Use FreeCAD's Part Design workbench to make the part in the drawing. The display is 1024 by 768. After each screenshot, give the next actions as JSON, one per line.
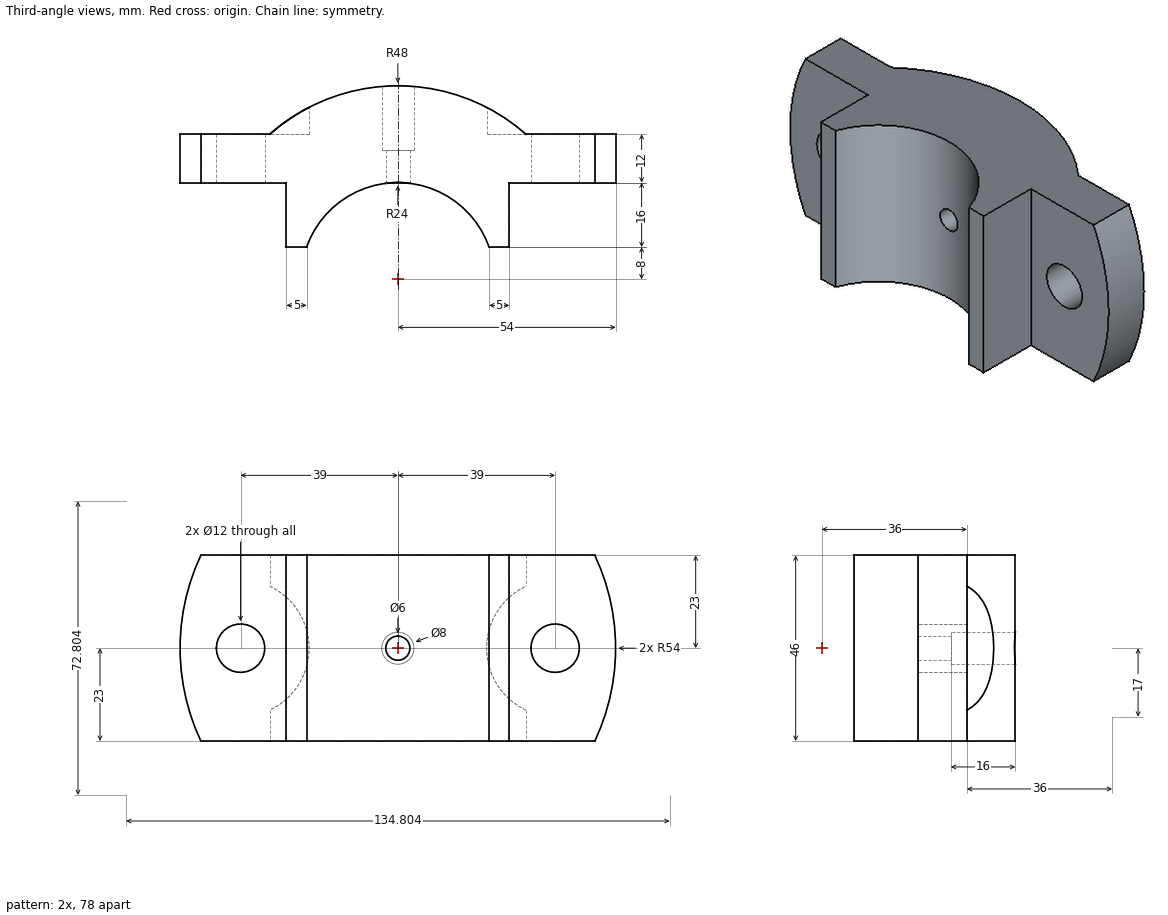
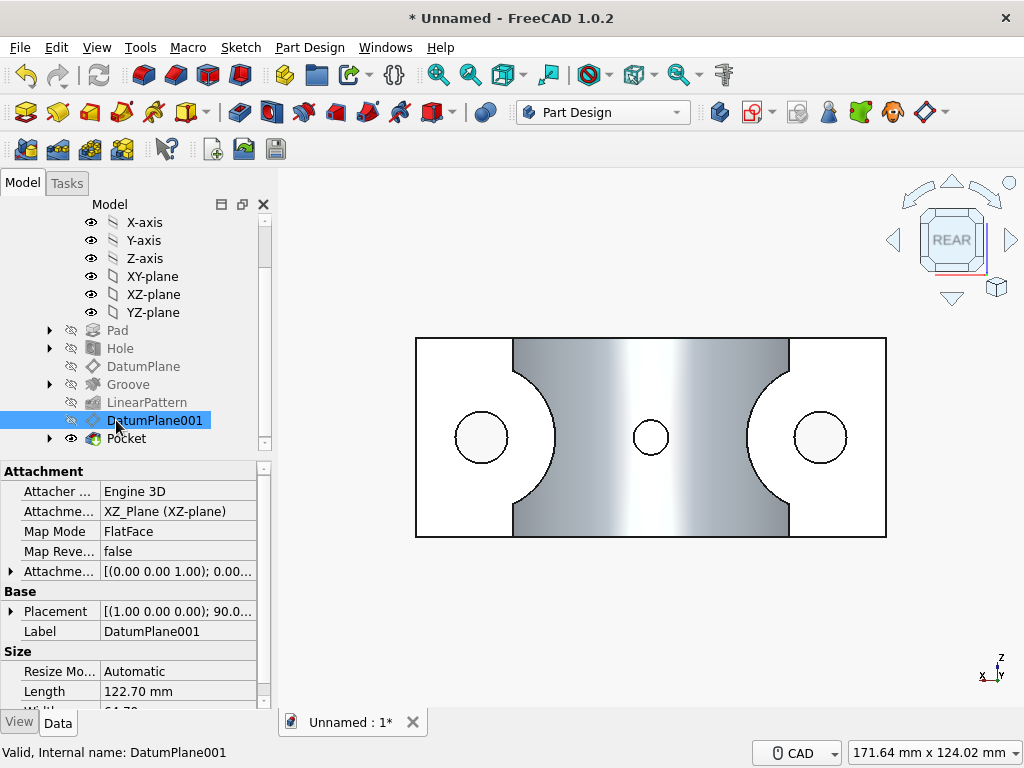
{"action": "scroll", "coordinate": [160, 326], "scroll_direction": "down", "scroll_amount": 3}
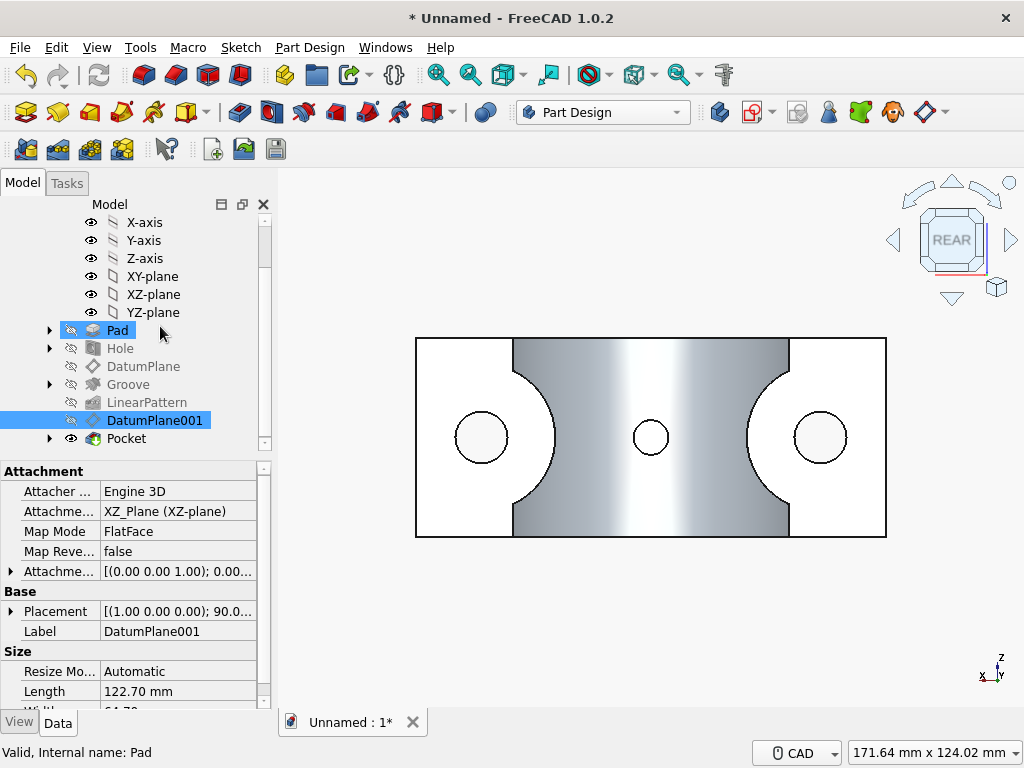
{"action": "scroll", "coordinate": [160, 326], "scroll_direction": "up", "scroll_amount": 15}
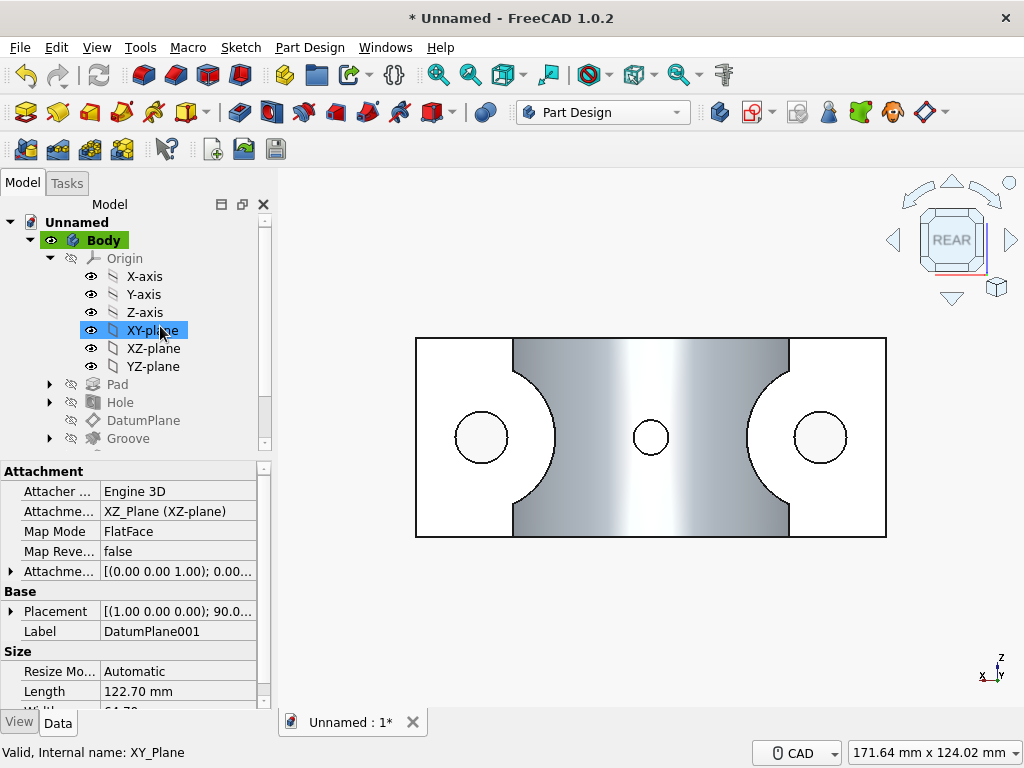
{"action": "left_click", "coordinate": [136, 348]}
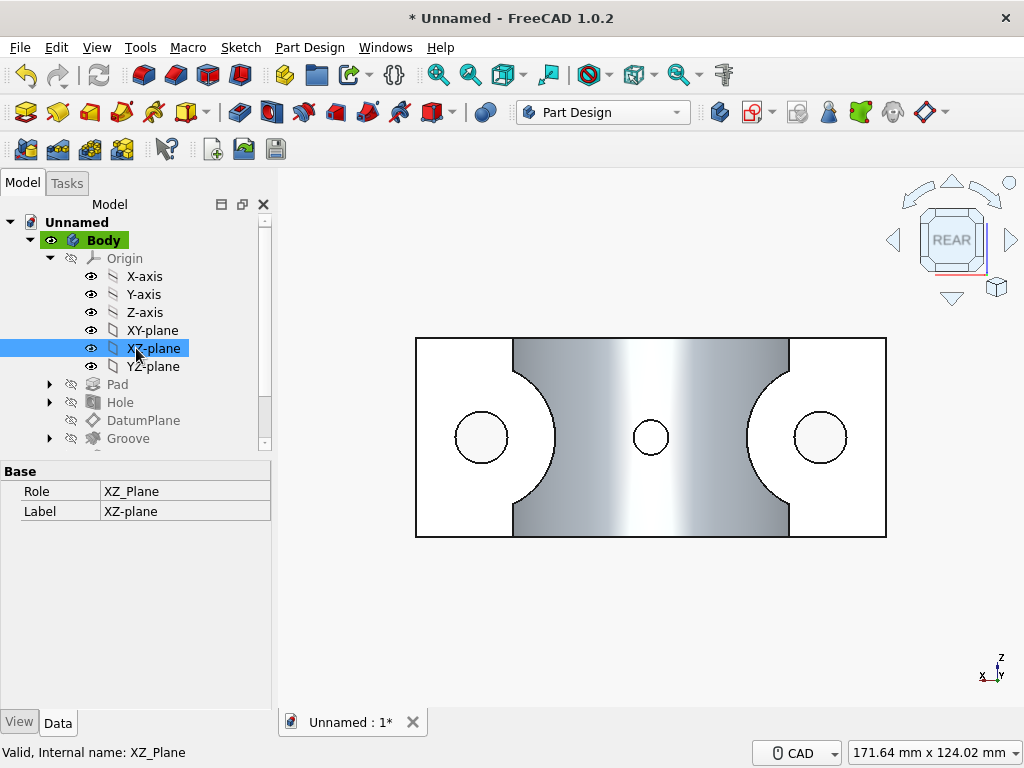
{"action": "left_click", "coordinate": [926, 112]}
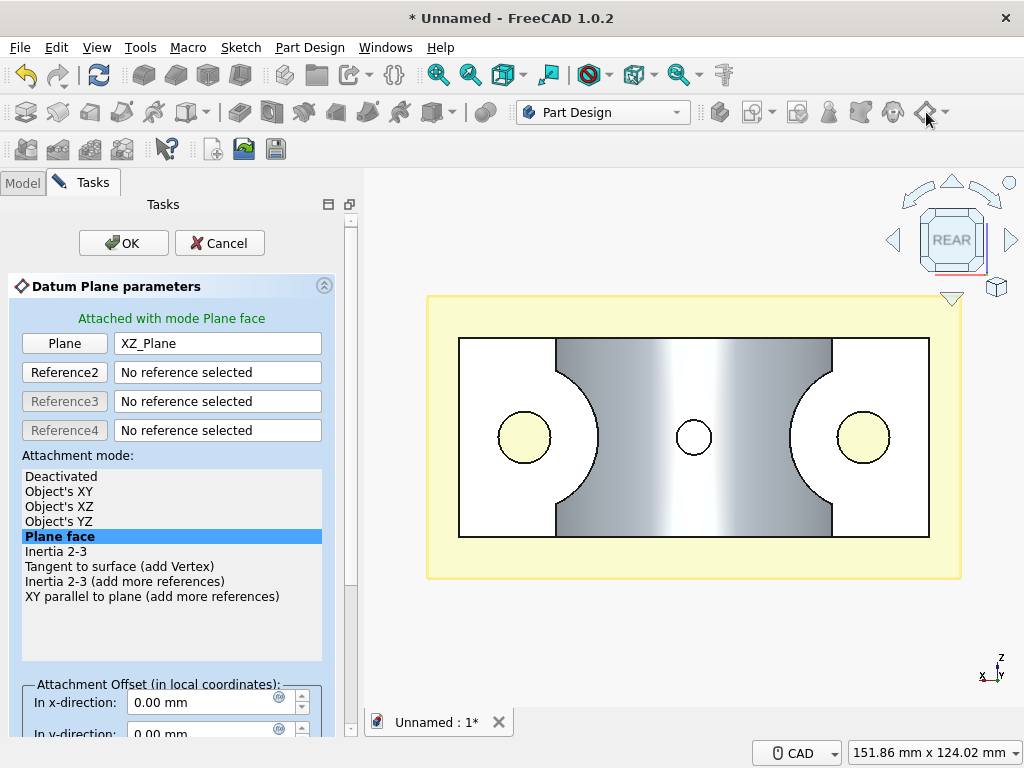
{"action": "scroll", "coordinate": [351, 475], "scroll_direction": "down", "scroll_amount": 2}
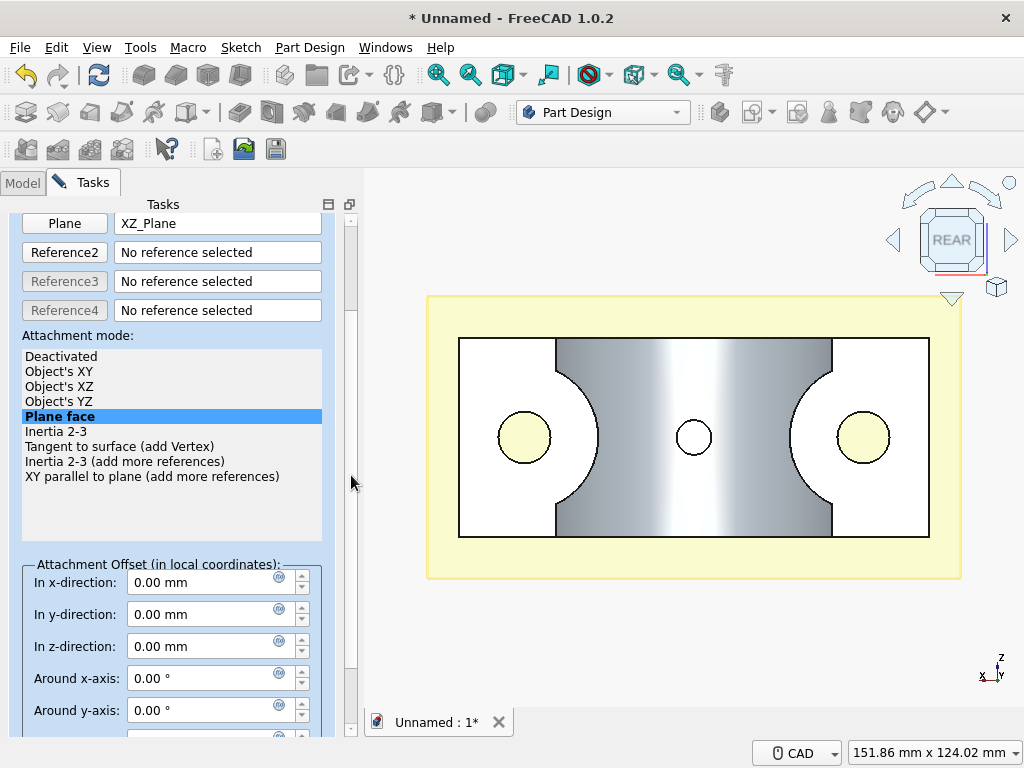
{"action": "triple_click", "coordinate": [210, 646]}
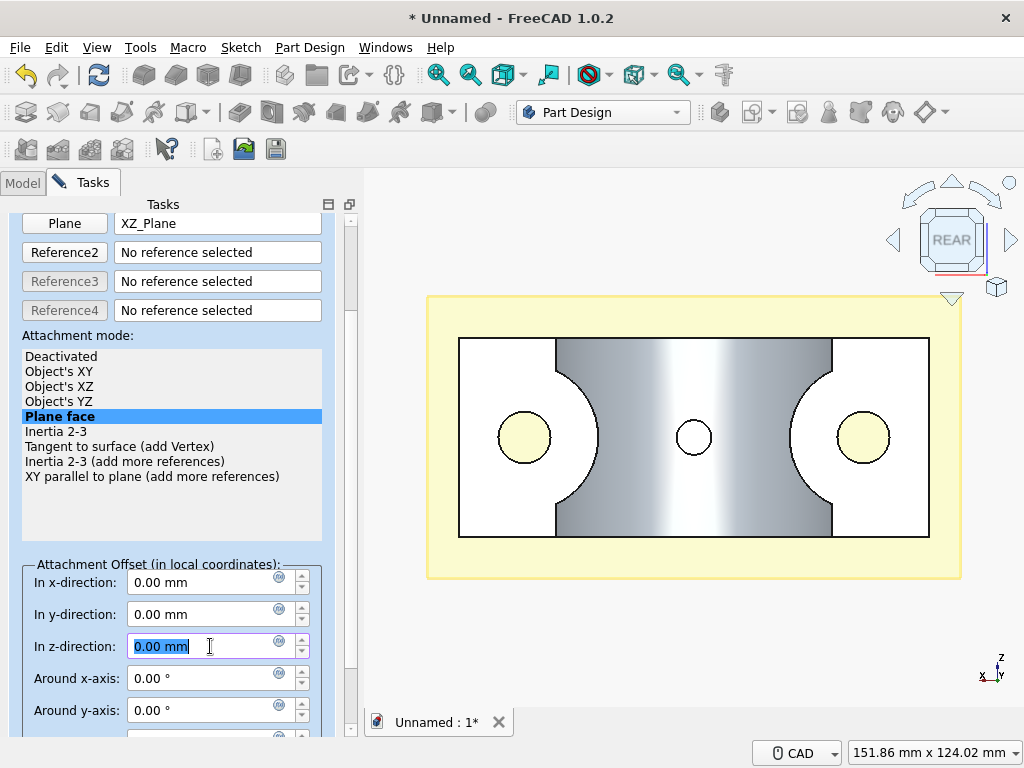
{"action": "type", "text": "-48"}
{"action": "key", "text": "Tab"}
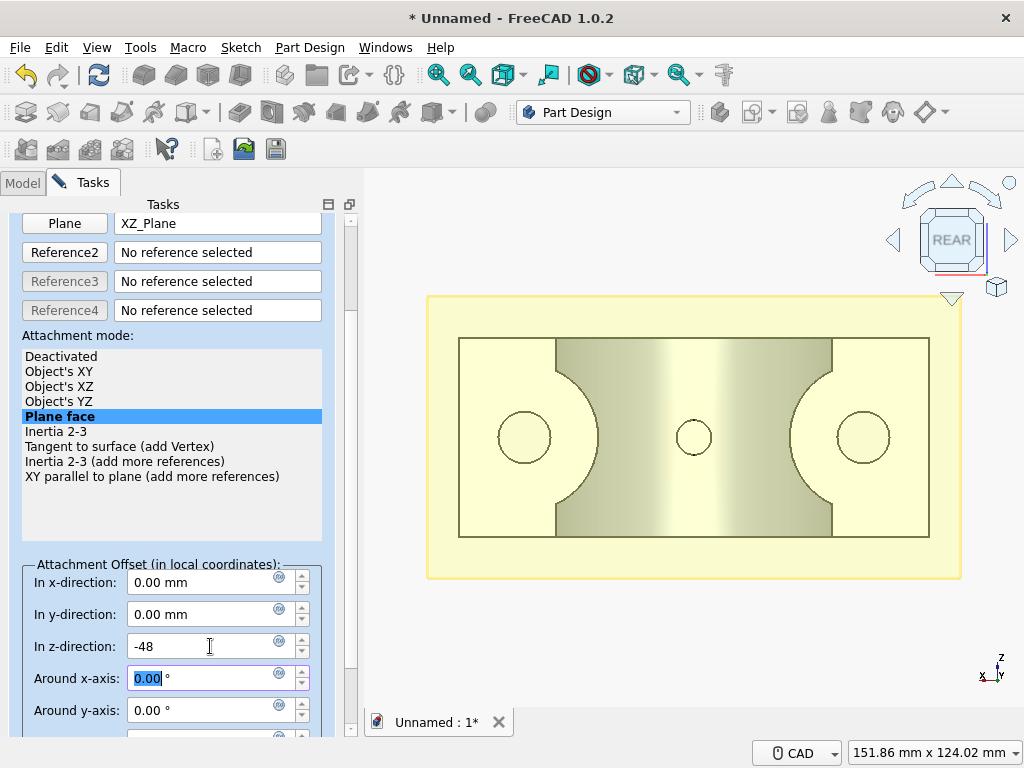
{"action": "scroll", "coordinate": [351, 475], "scroll_direction": "up", "scroll_amount": 3}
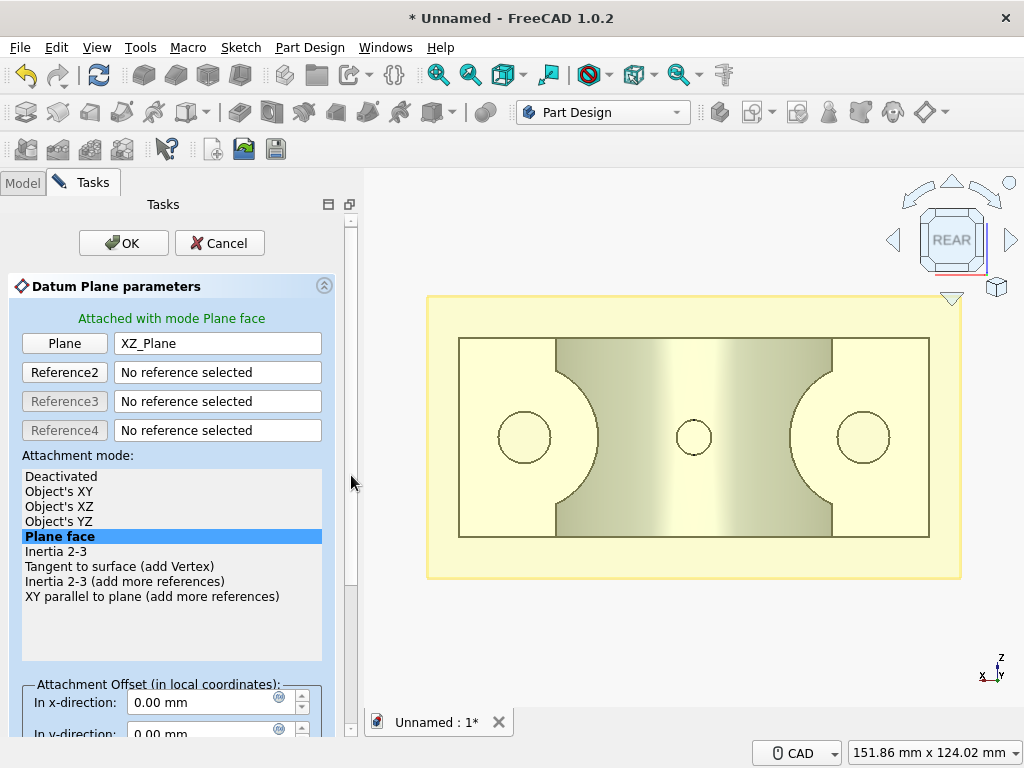
{"action": "left_click", "coordinate": [124, 243]}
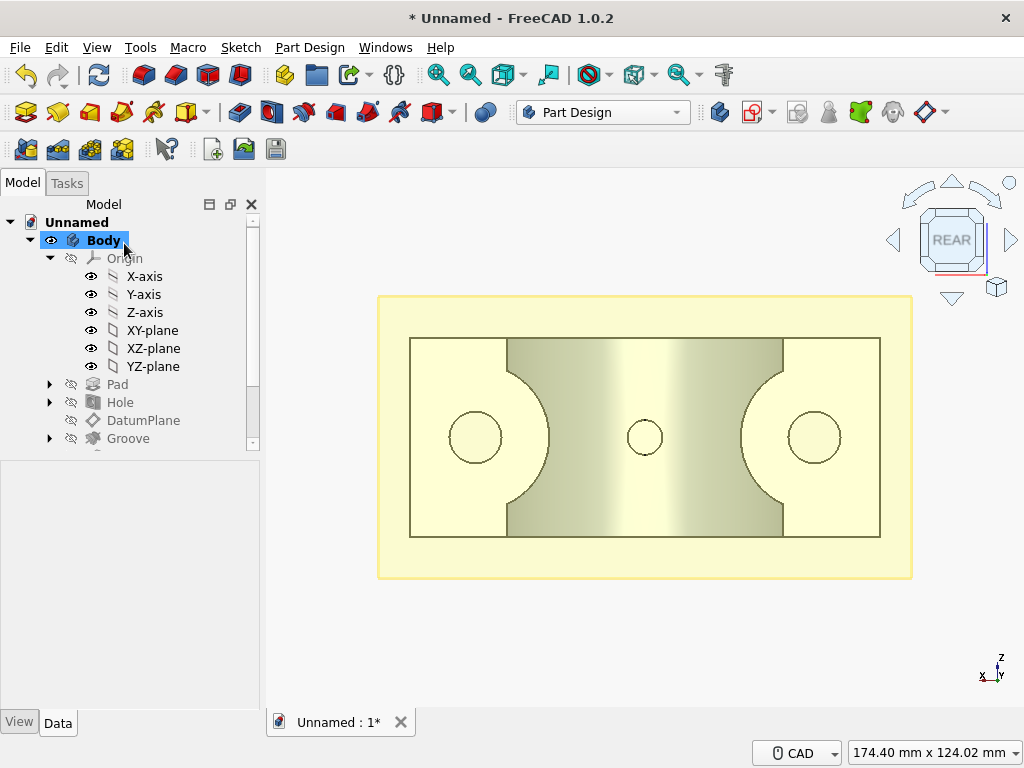
{"action": "scroll", "coordinate": [100, 326], "scroll_direction": "down", "scroll_amount": 3}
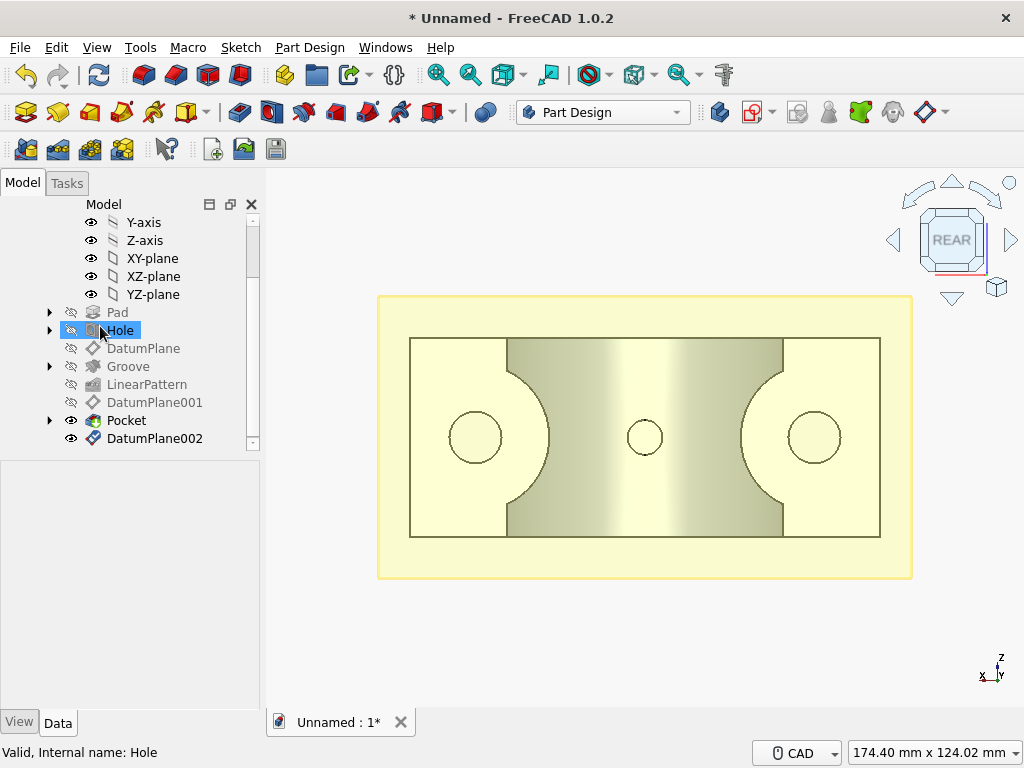
{"action": "left_click", "coordinate": [116, 438]}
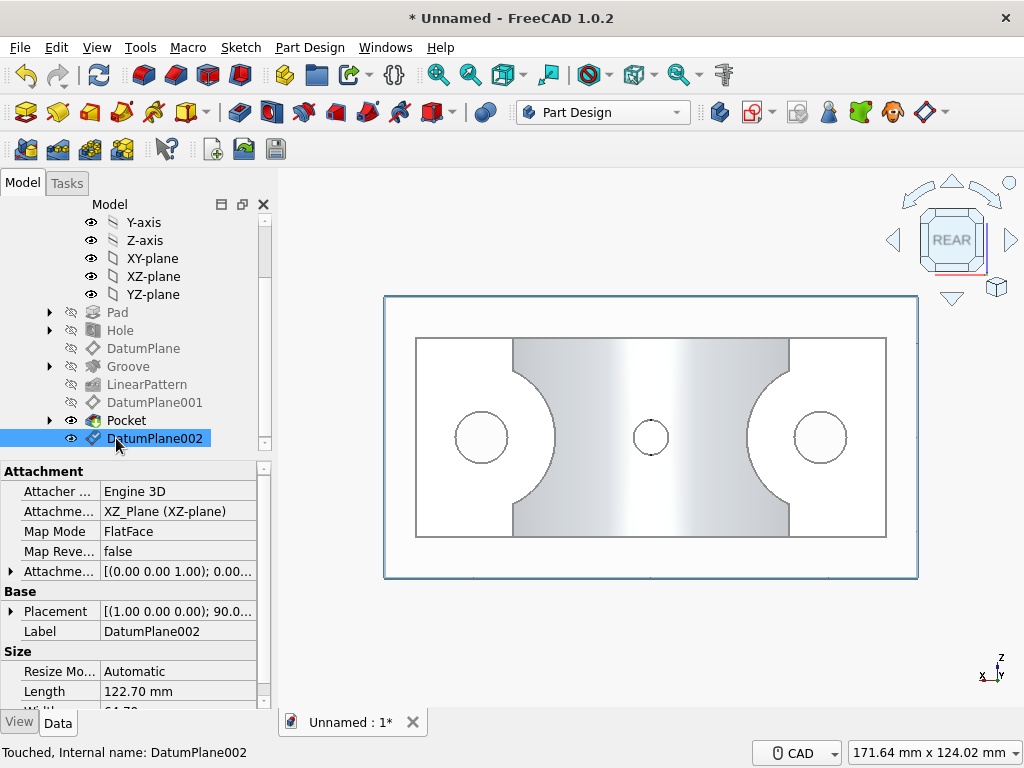
{"action": "left_click", "coordinate": [752, 112]}